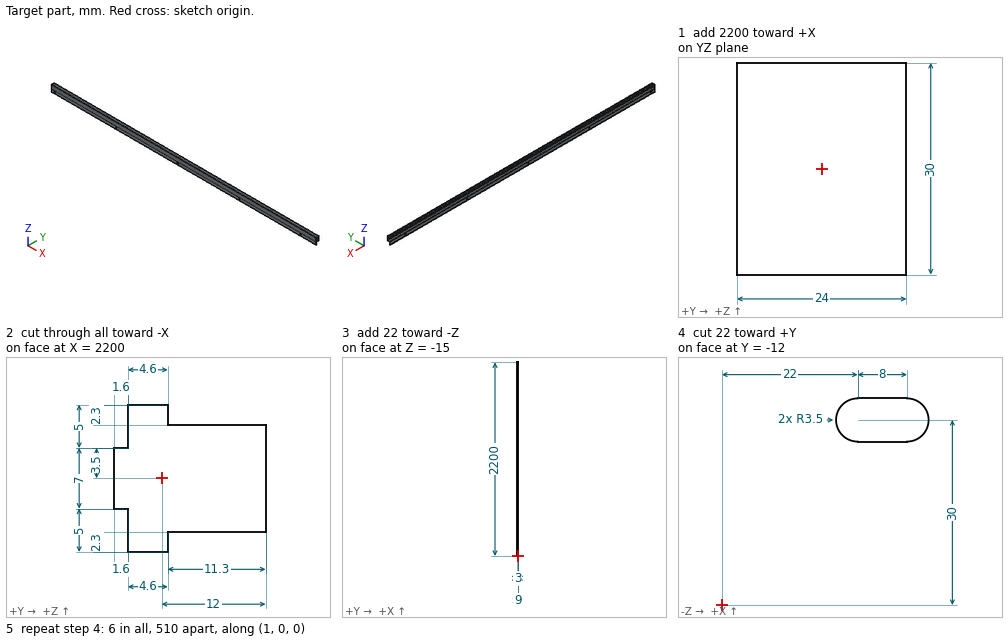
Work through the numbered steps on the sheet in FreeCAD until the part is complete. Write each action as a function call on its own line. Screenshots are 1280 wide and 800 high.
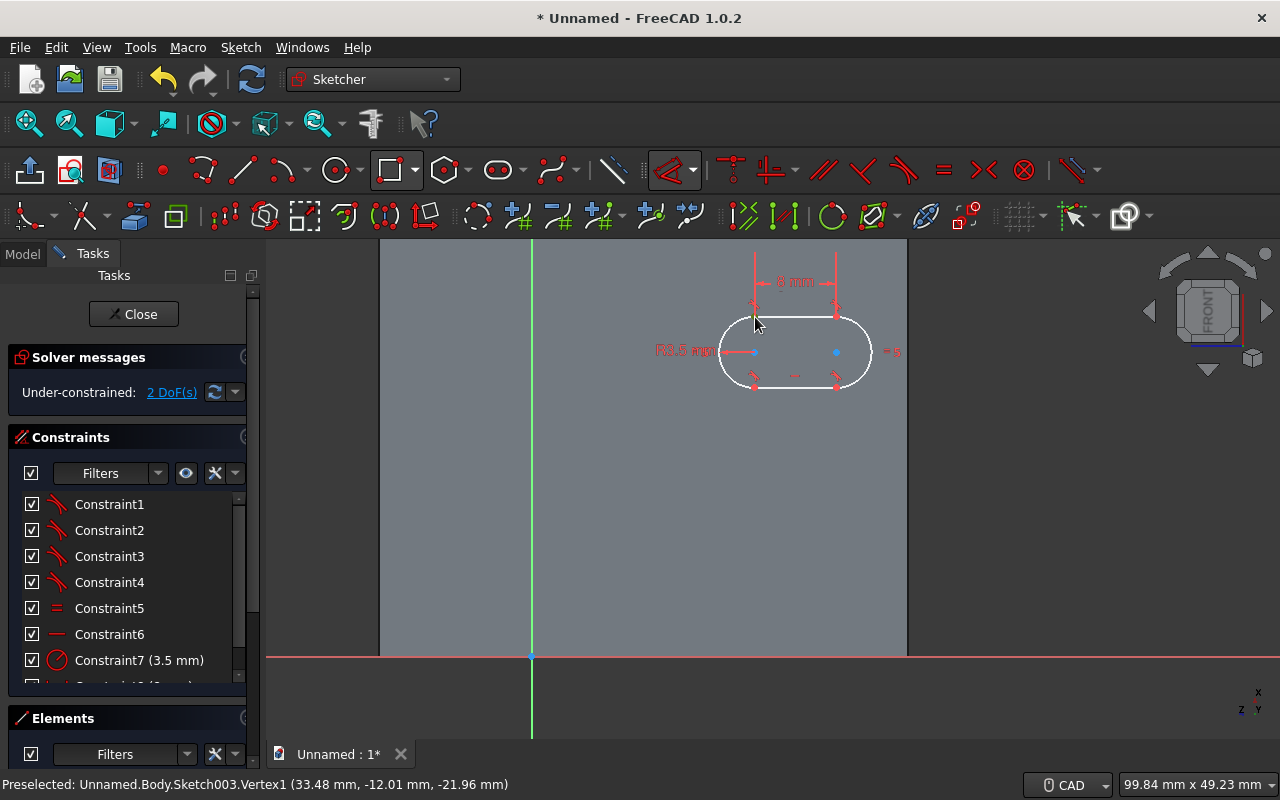
key(l)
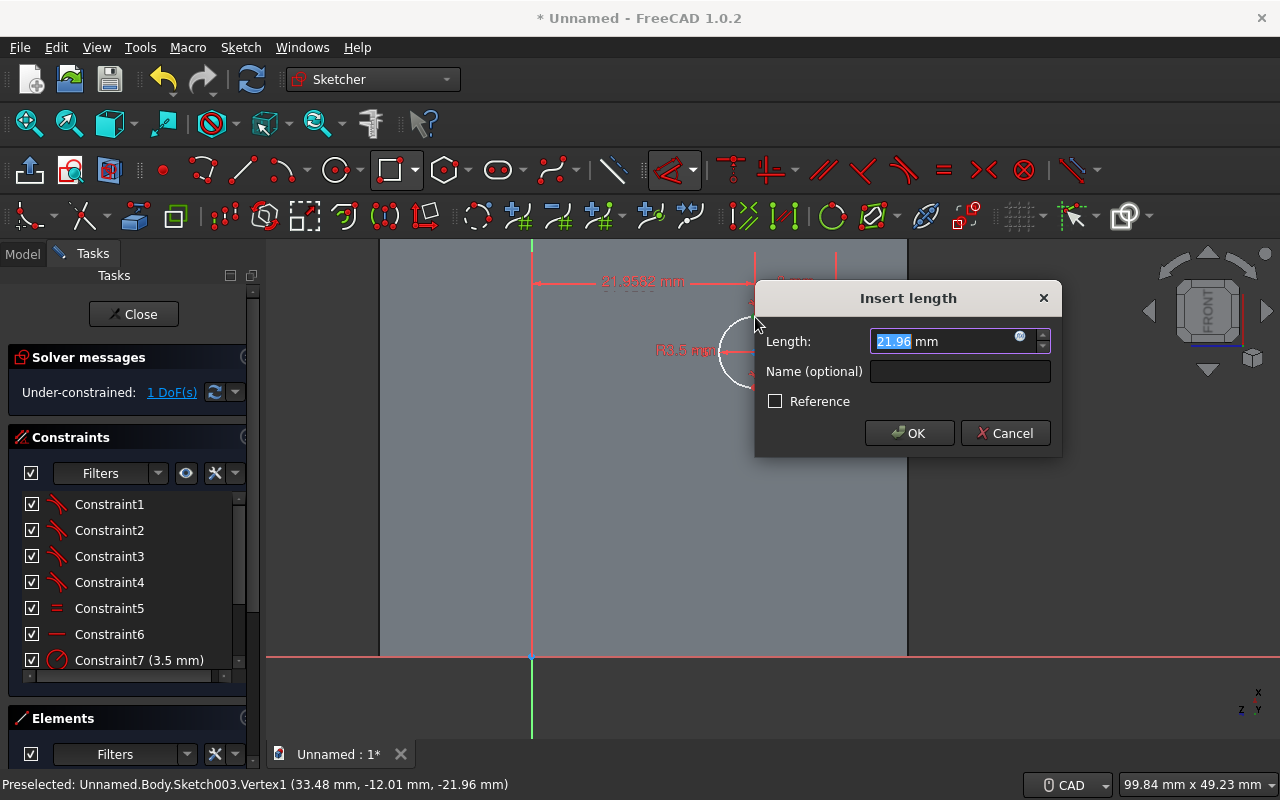
text(22)
key(Return)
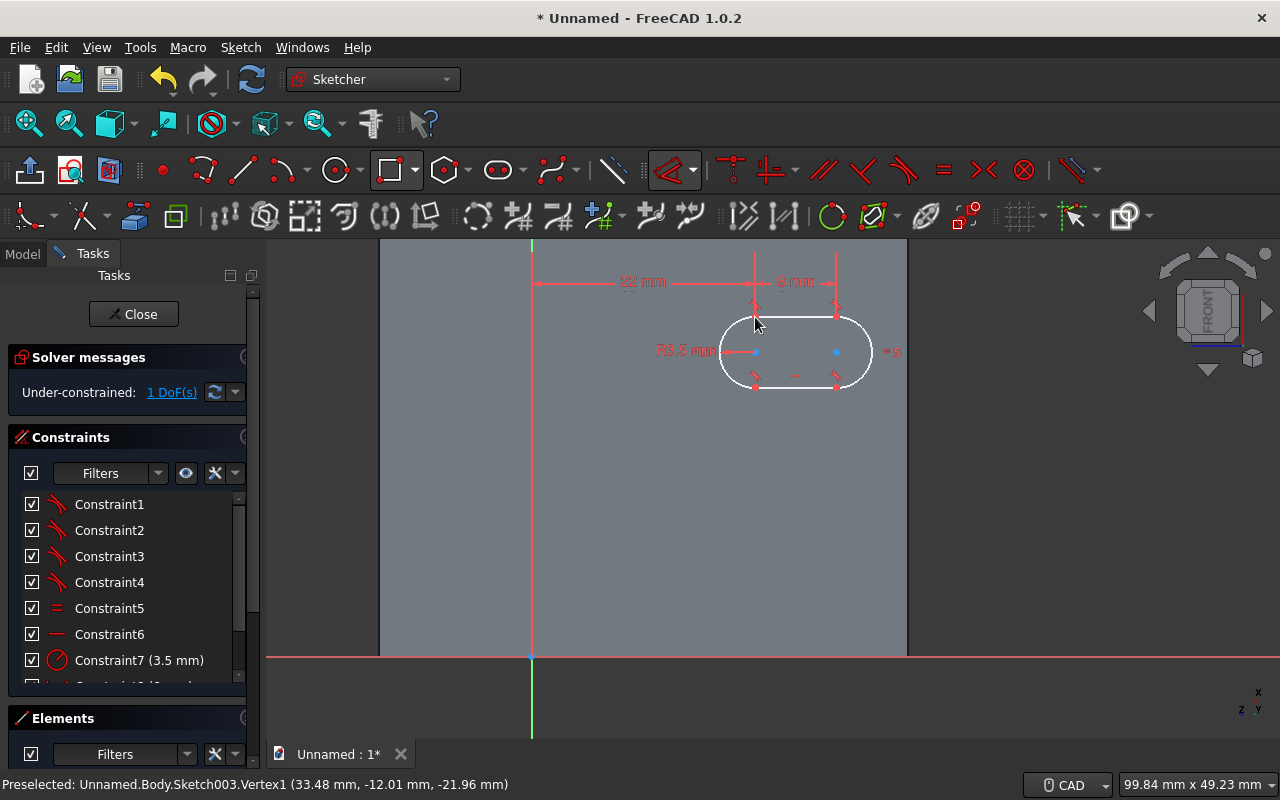
click(755, 352)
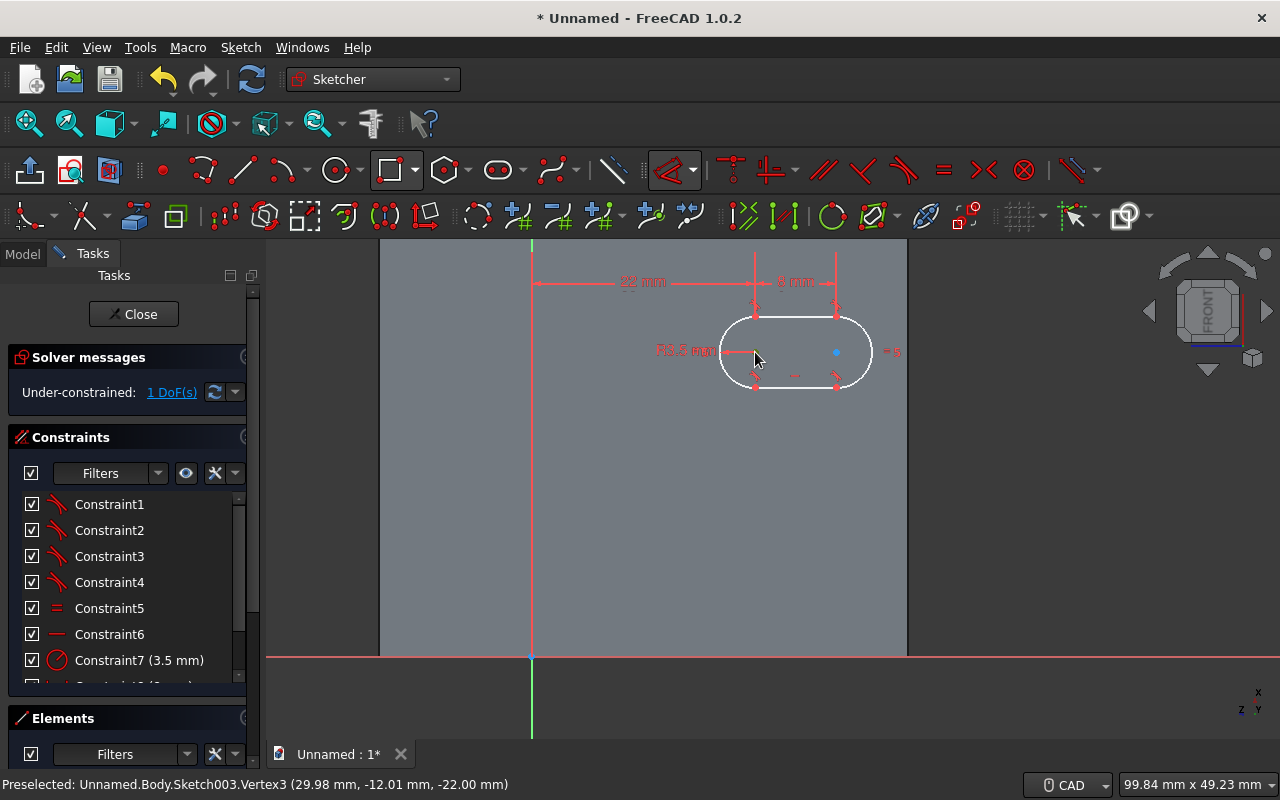
click(696, 170)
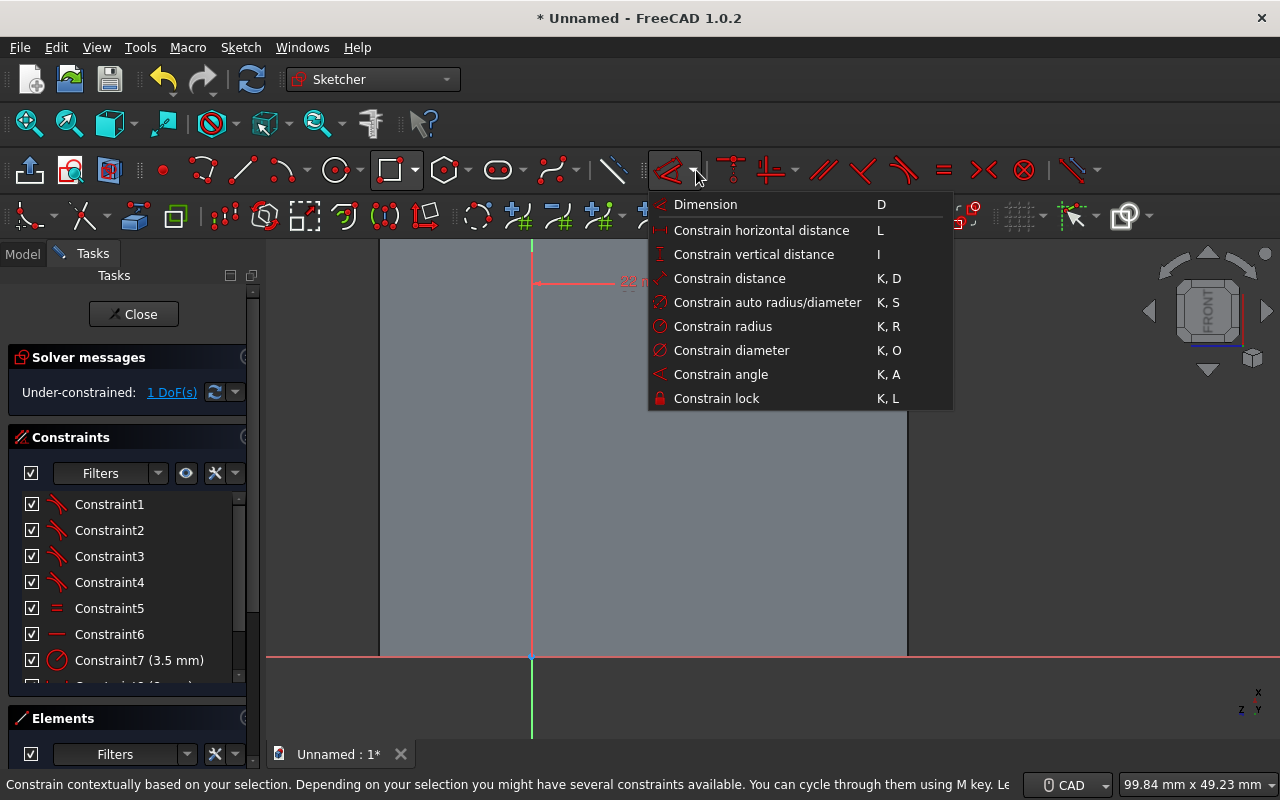
click(801, 254)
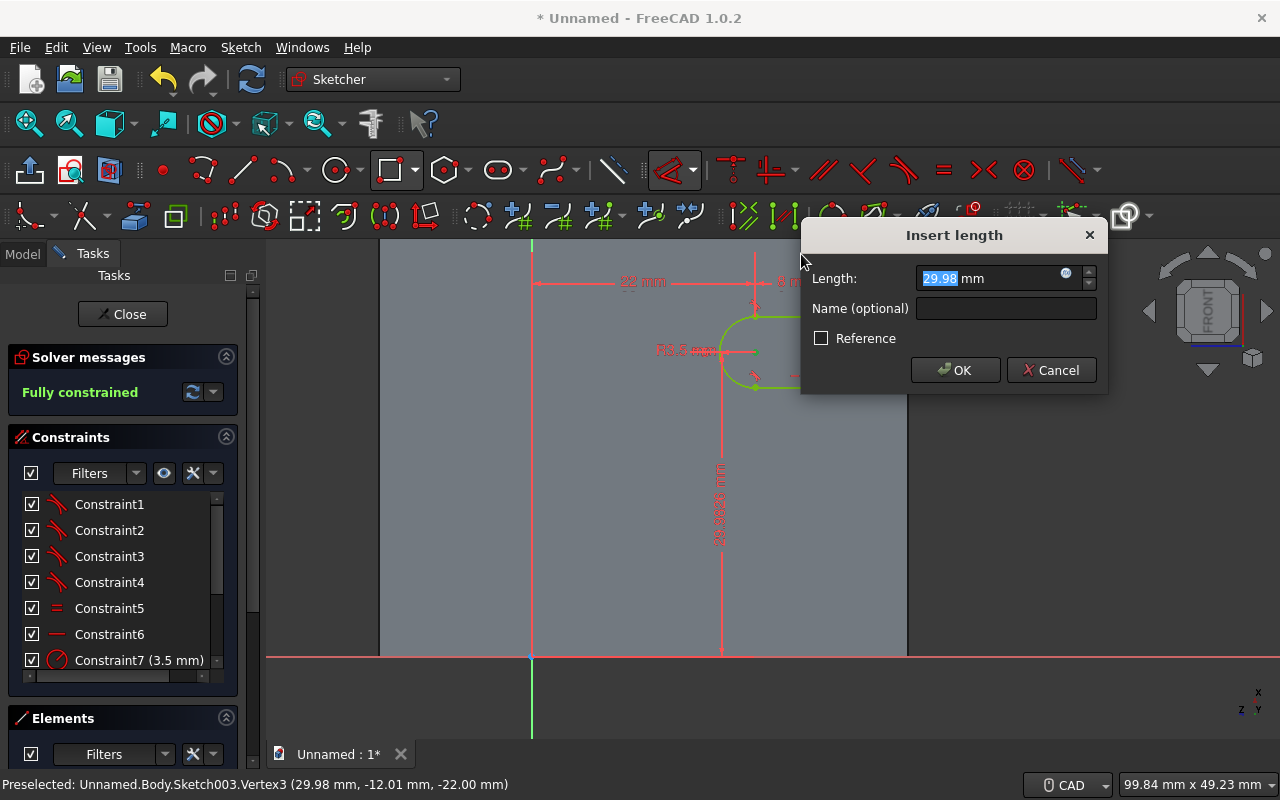
text(30)
key(Return)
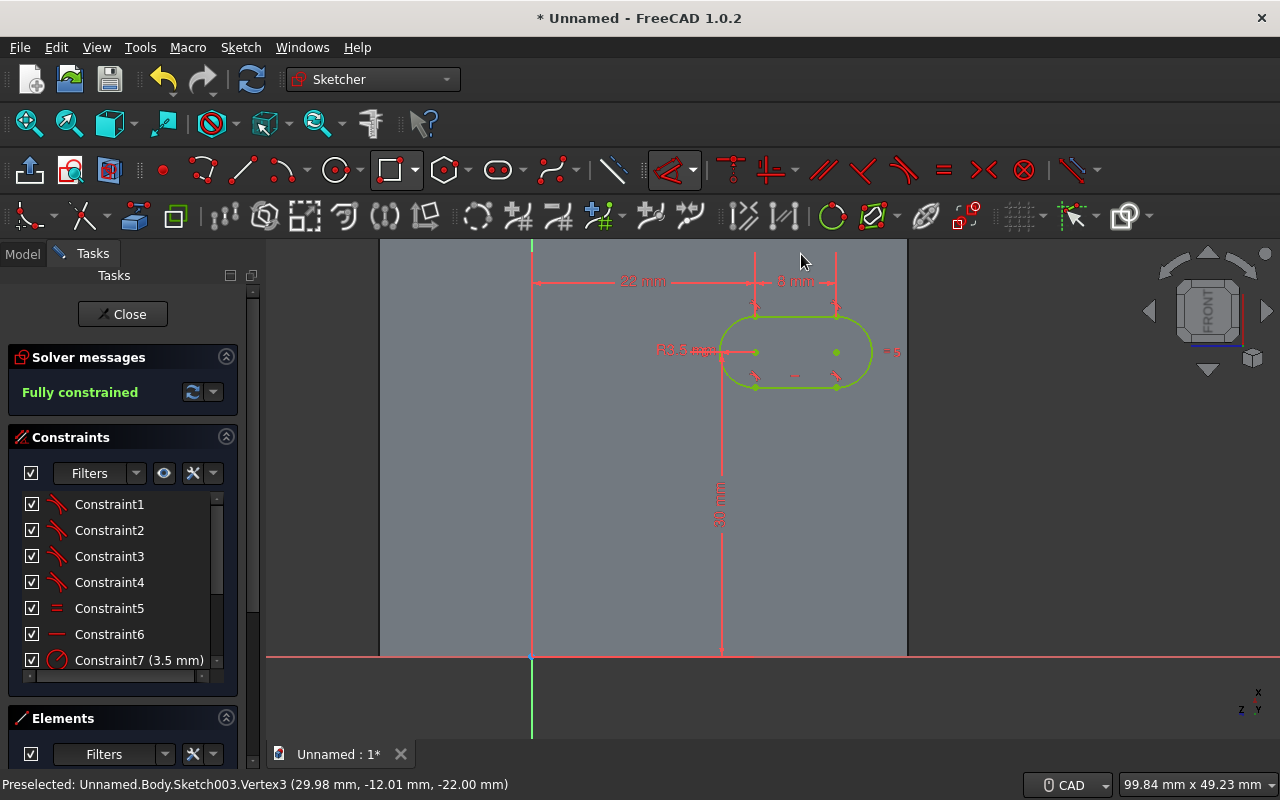
click(123, 314)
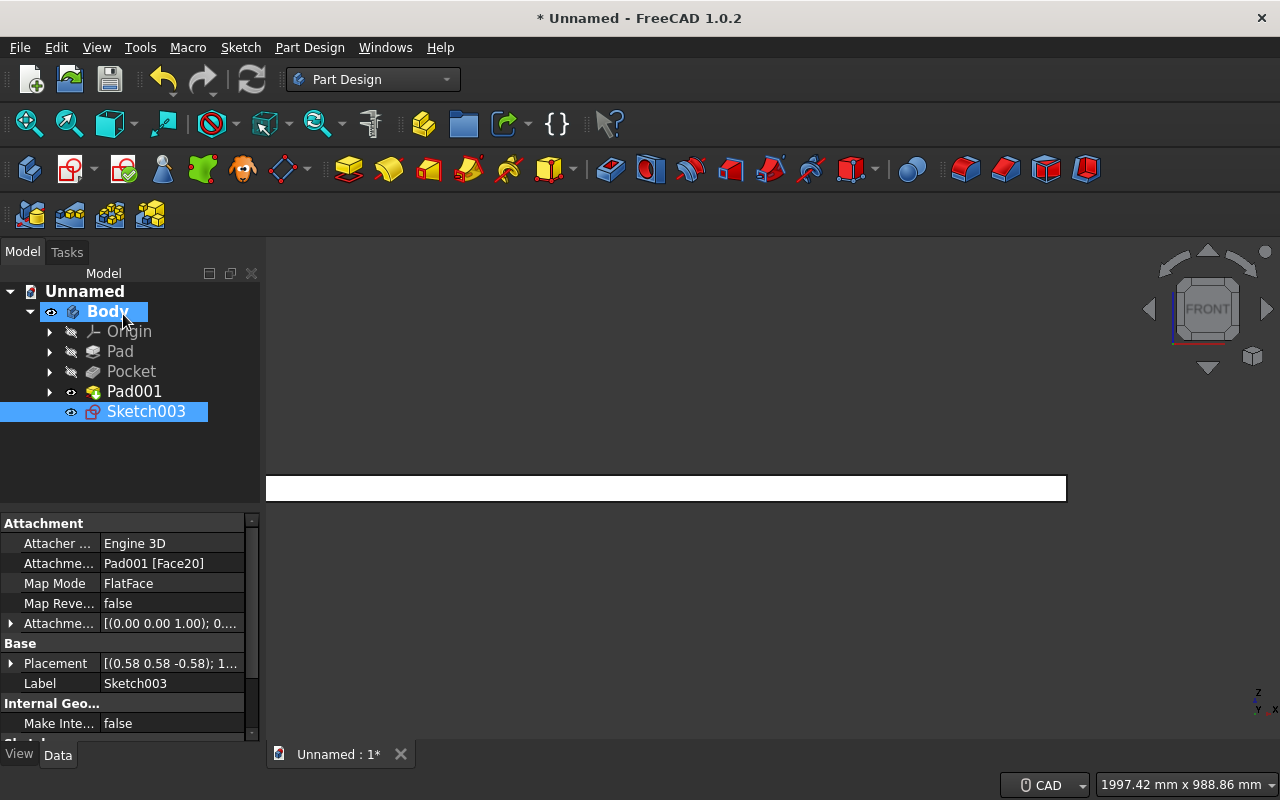
click(612, 170)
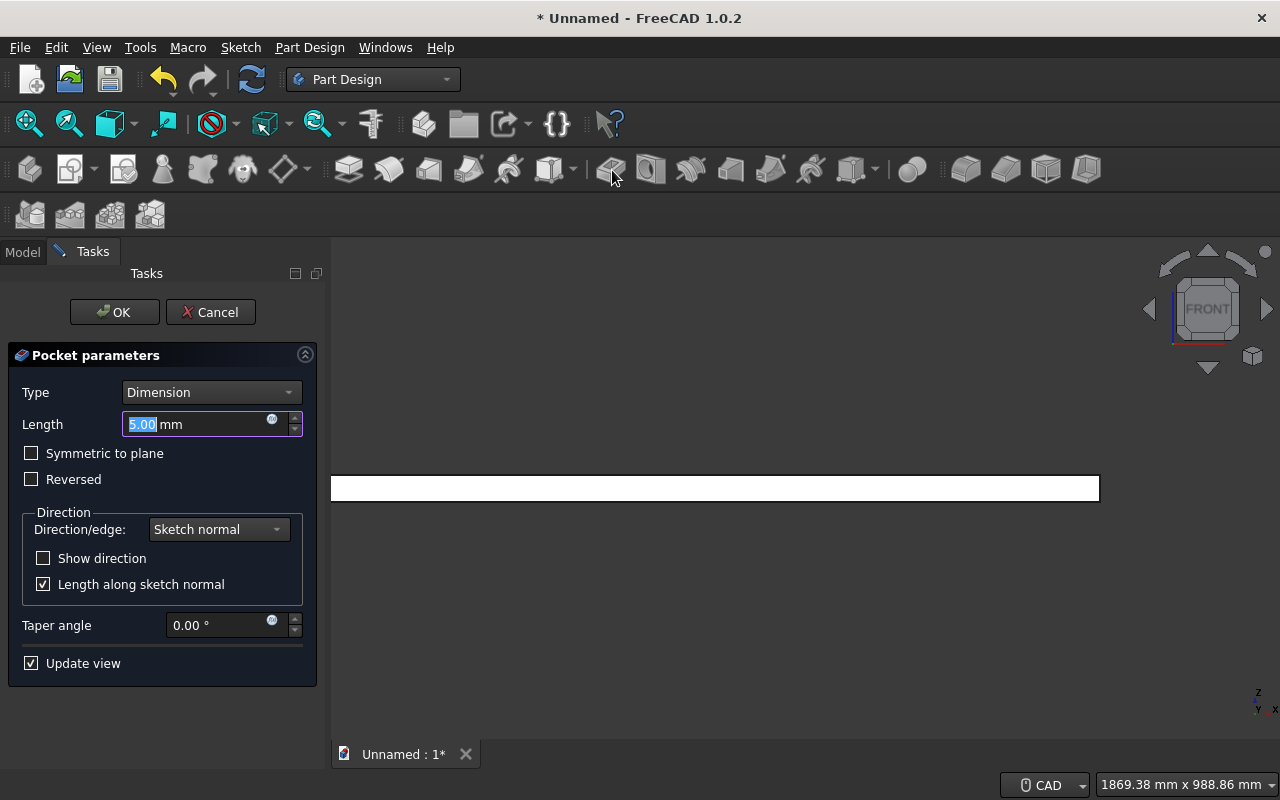
text(22)
key(Tab)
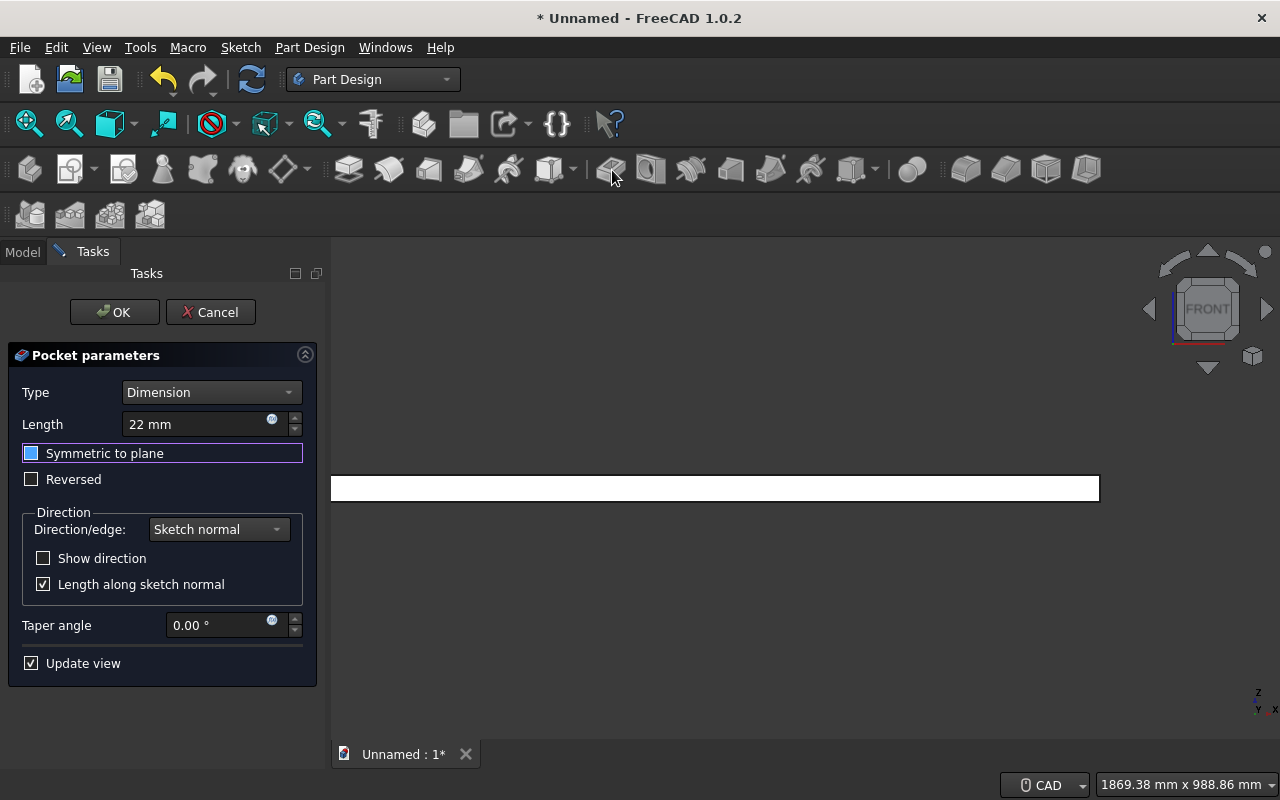
click(115, 312)